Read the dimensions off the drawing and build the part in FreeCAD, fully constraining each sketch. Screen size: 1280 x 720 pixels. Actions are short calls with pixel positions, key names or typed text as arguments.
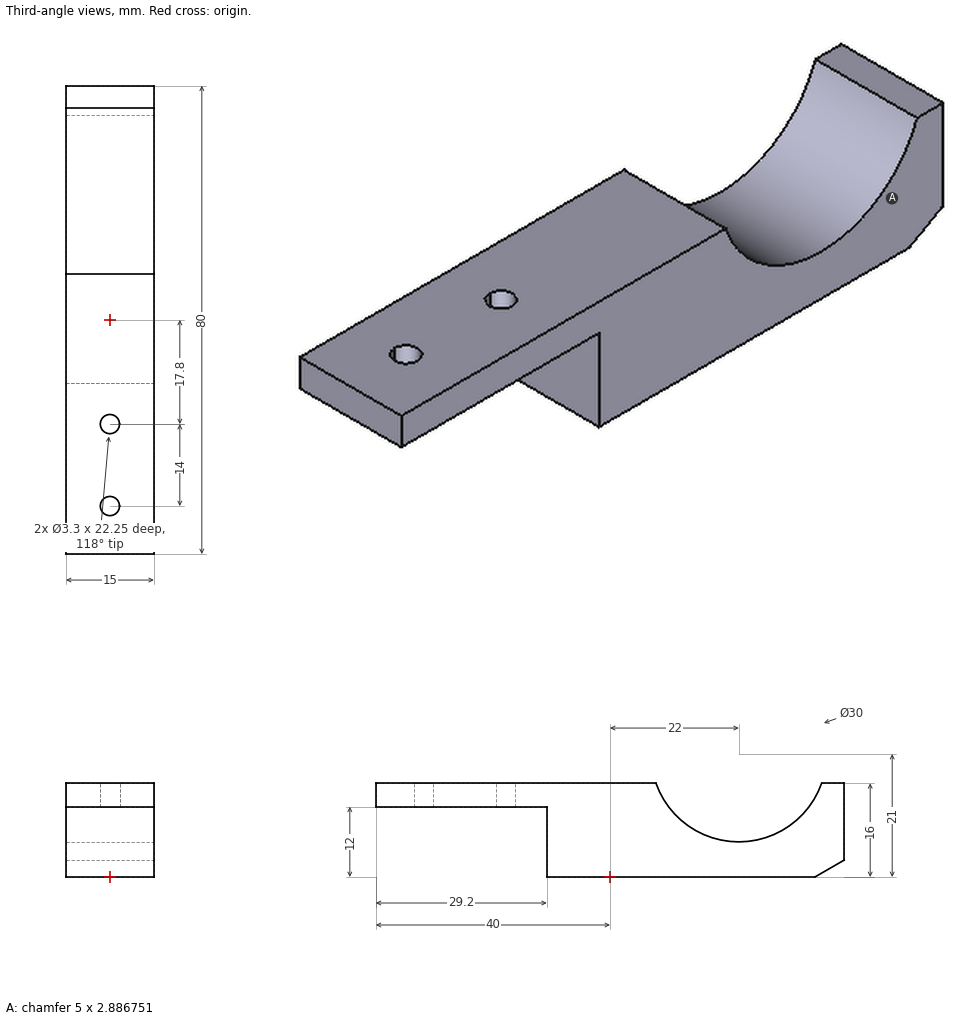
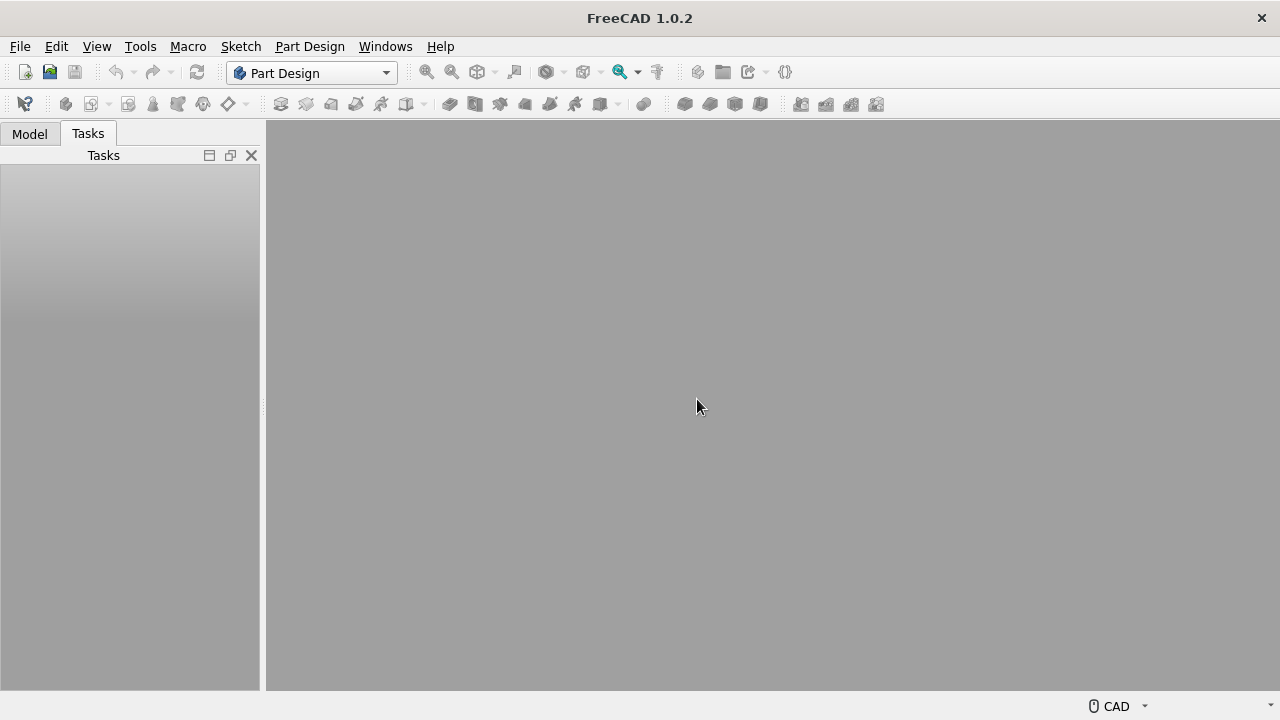
click(25, 72)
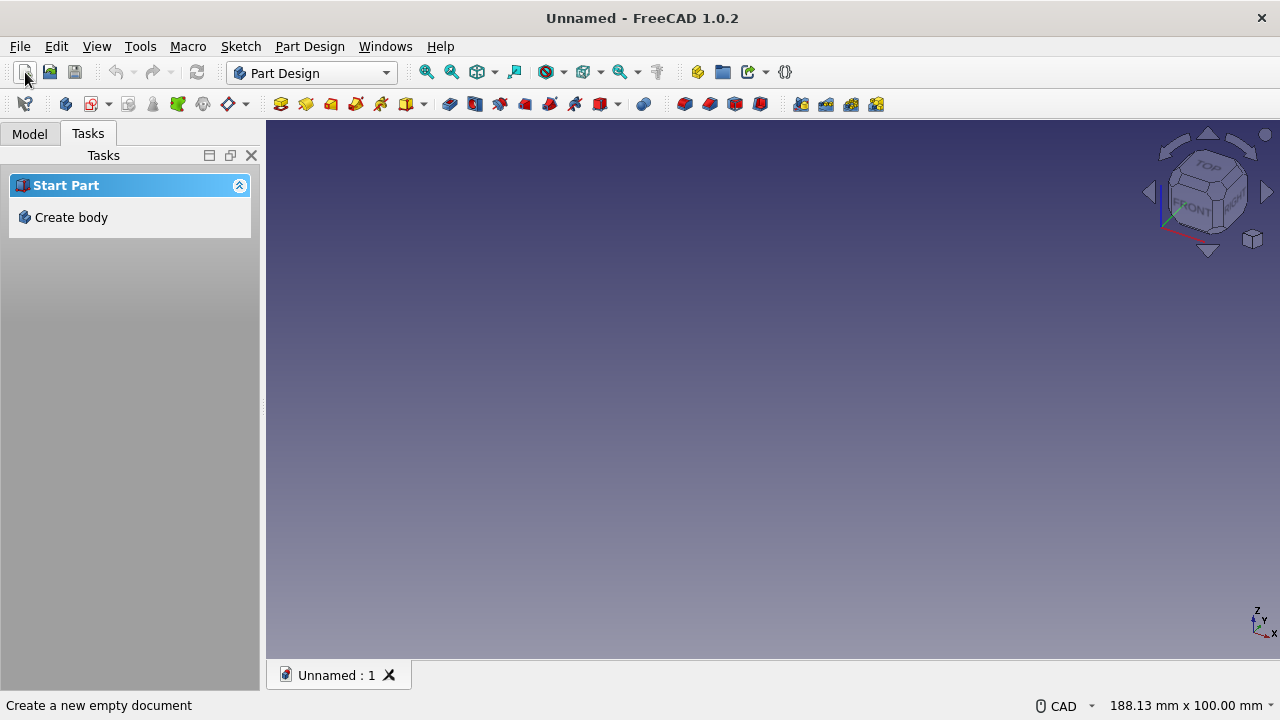
click(90, 104)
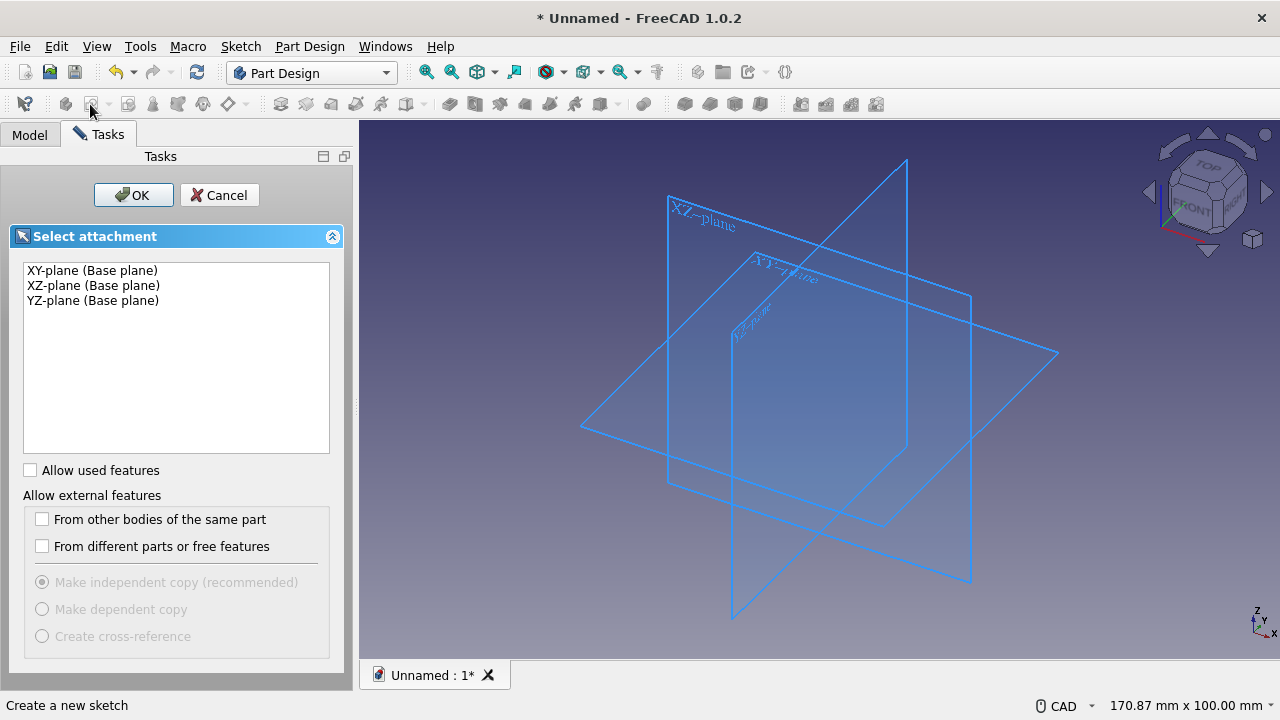
click(84, 270)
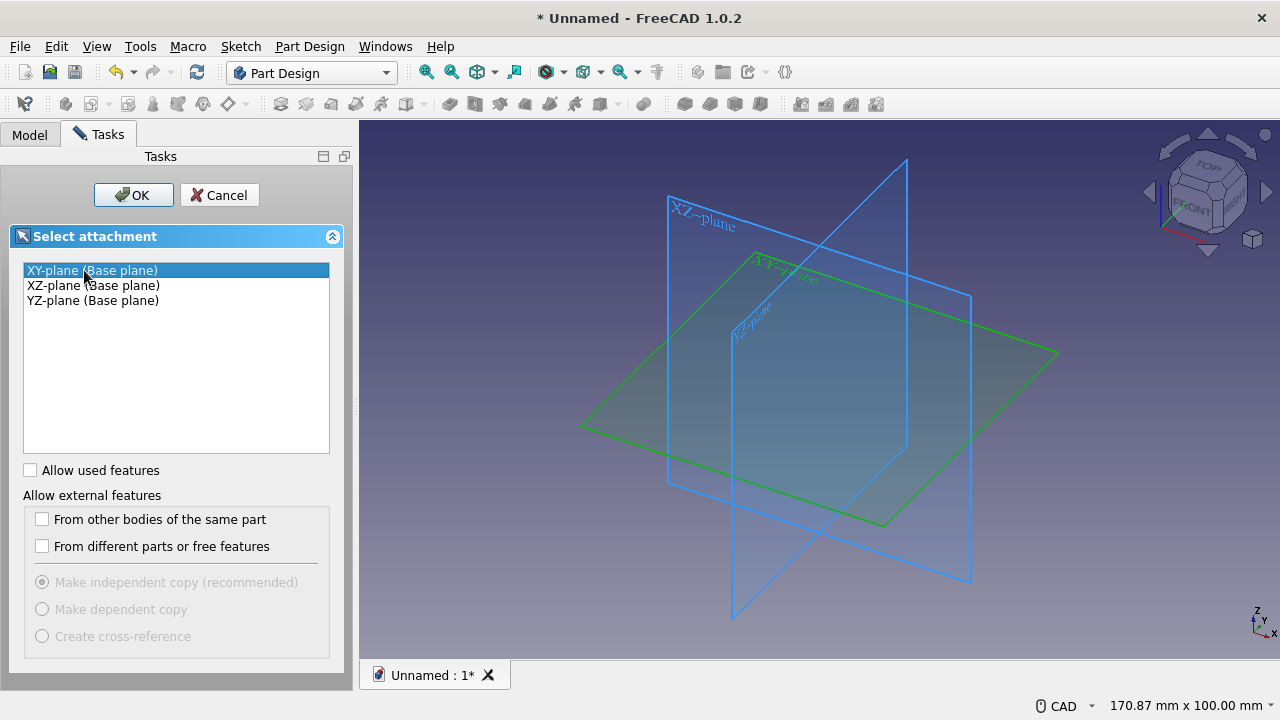
click(134, 195)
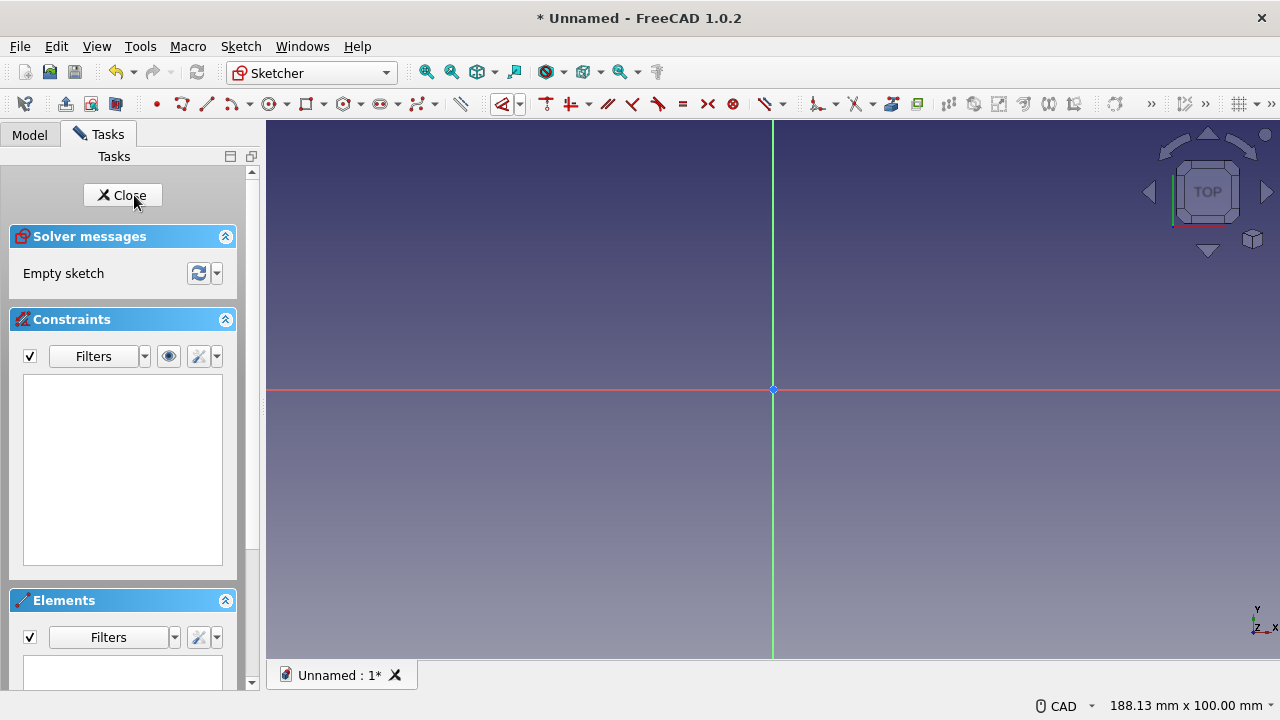
click(324, 104)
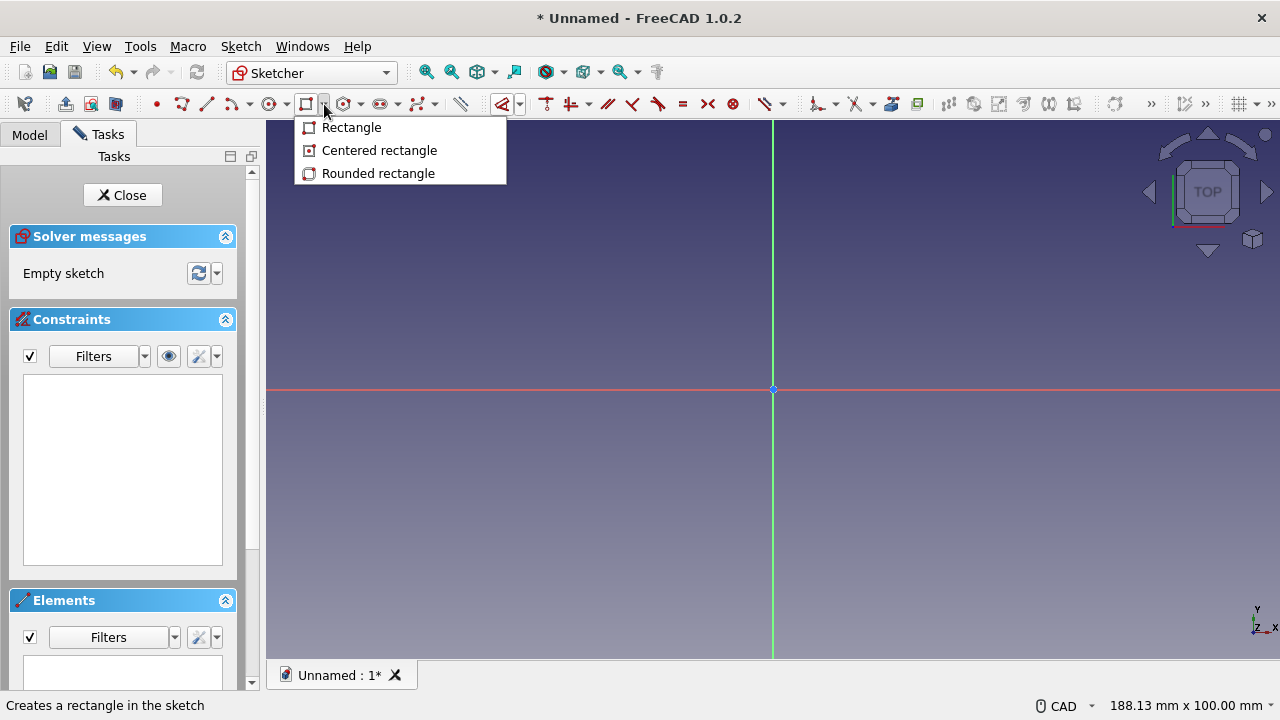
click(400, 150)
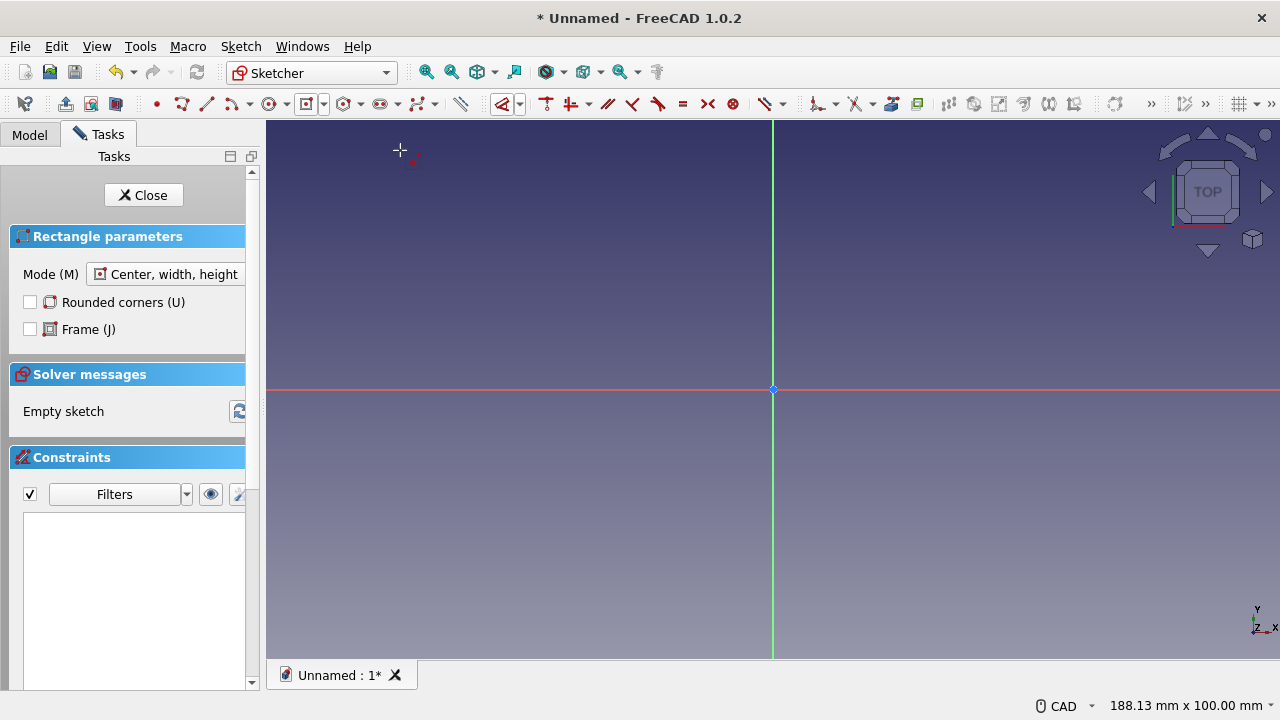
click(773, 390)
click(813, 174)
key(Escape)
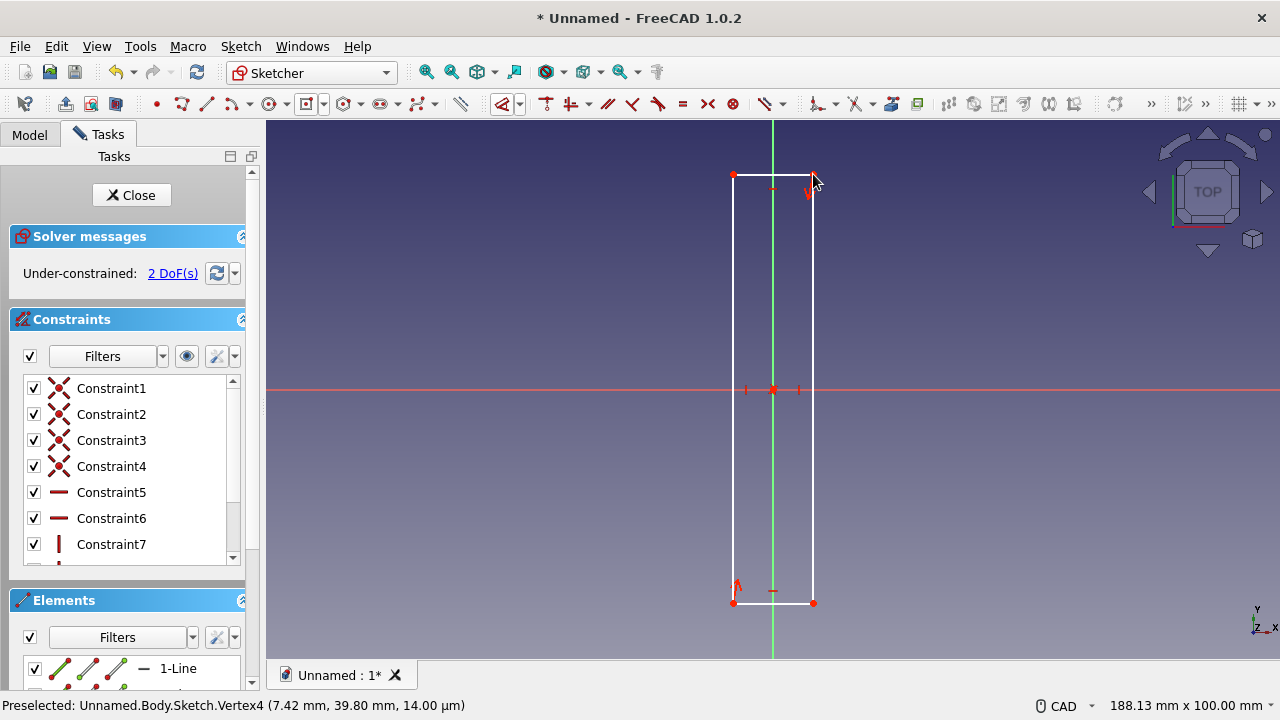
click(502, 104)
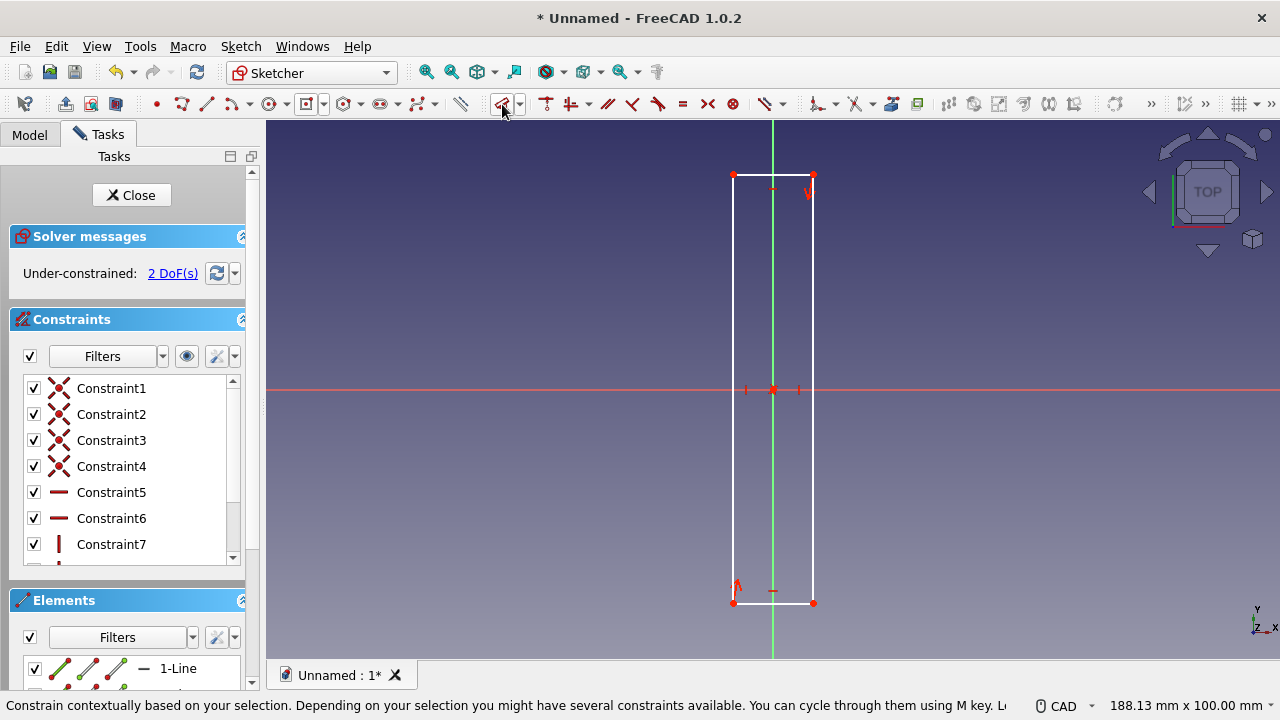
click(757, 604)
click(755, 570)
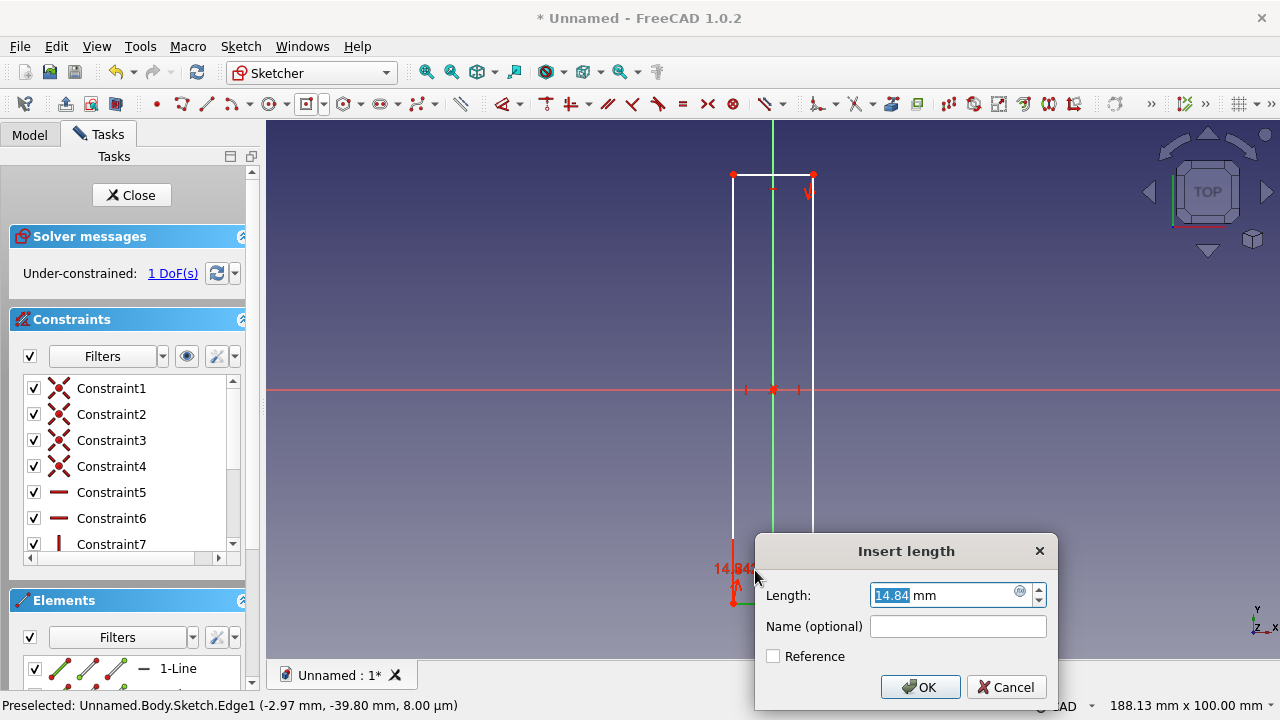
text(15)
key(Return)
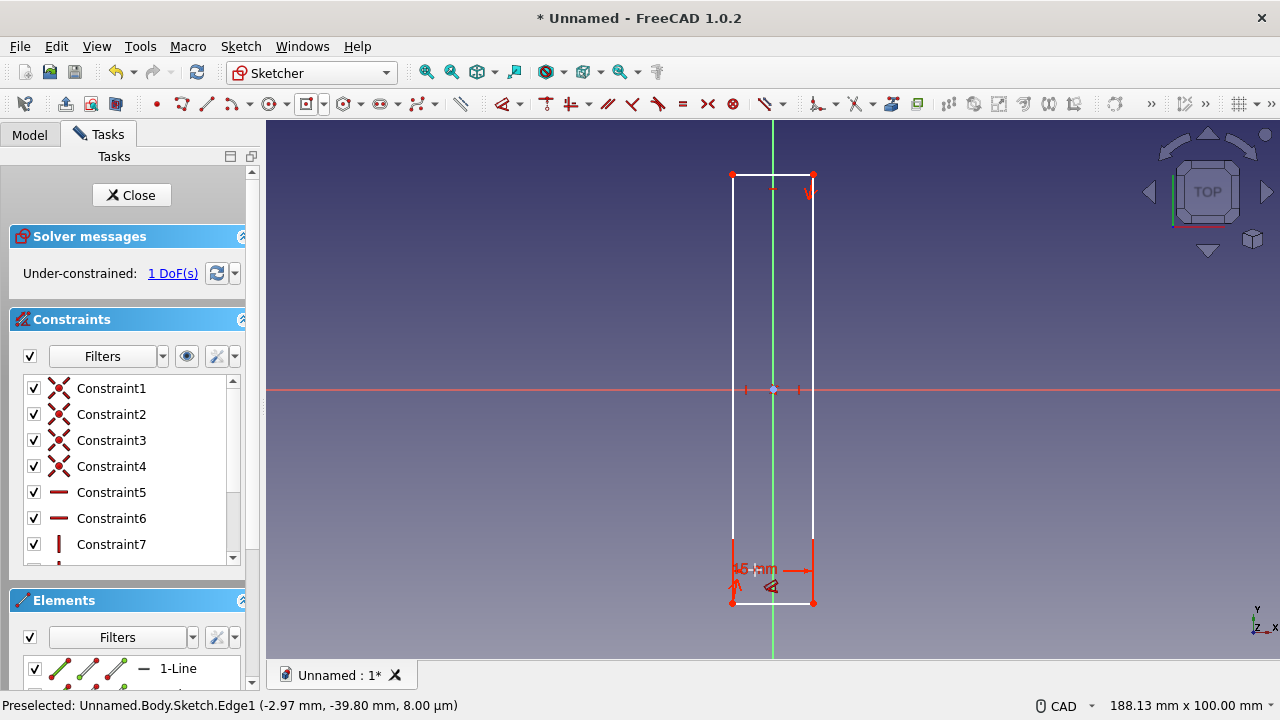
click(813, 475)
click(847, 291)